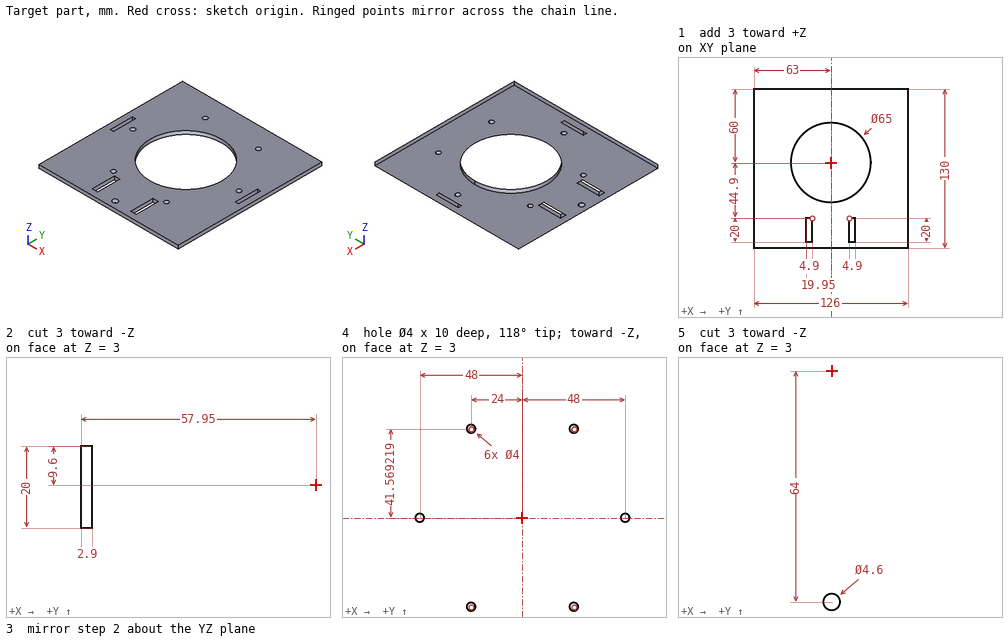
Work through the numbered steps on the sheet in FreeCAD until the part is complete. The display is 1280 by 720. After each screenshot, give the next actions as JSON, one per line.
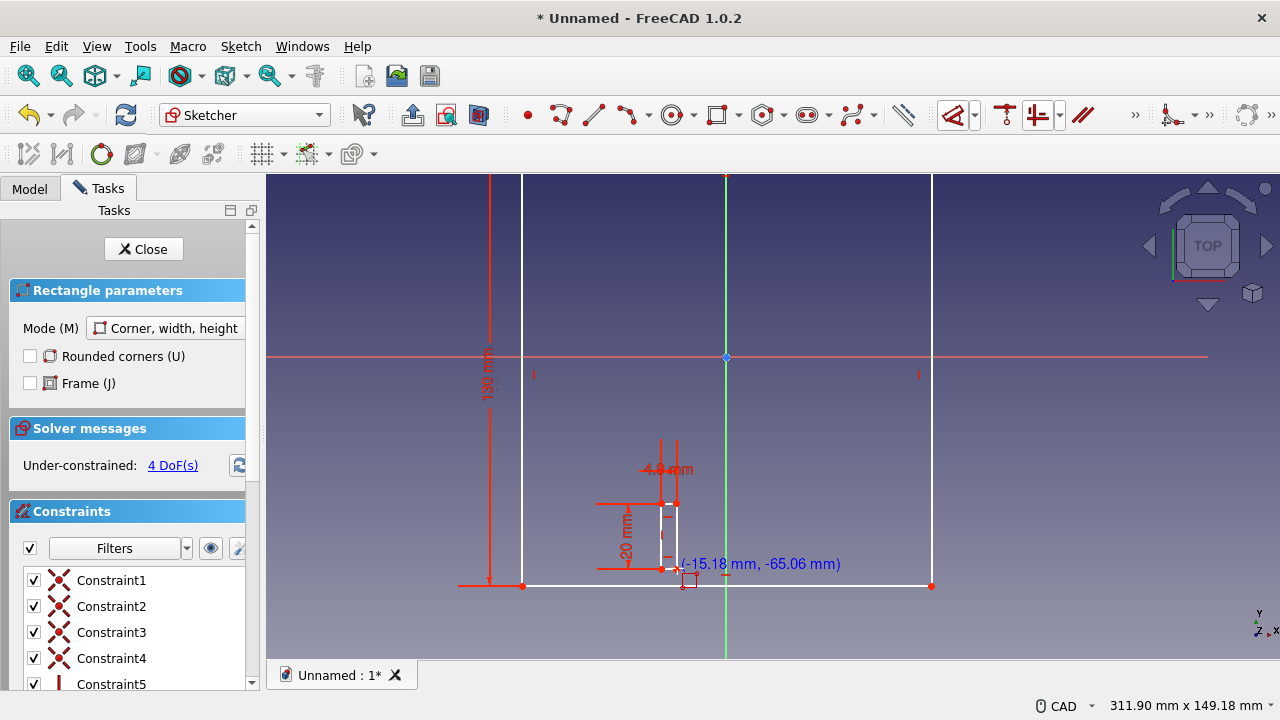
{"action": "left_click", "coordinate": [775, 503]}
{"action": "mouse_move", "coordinate": [791, 568]}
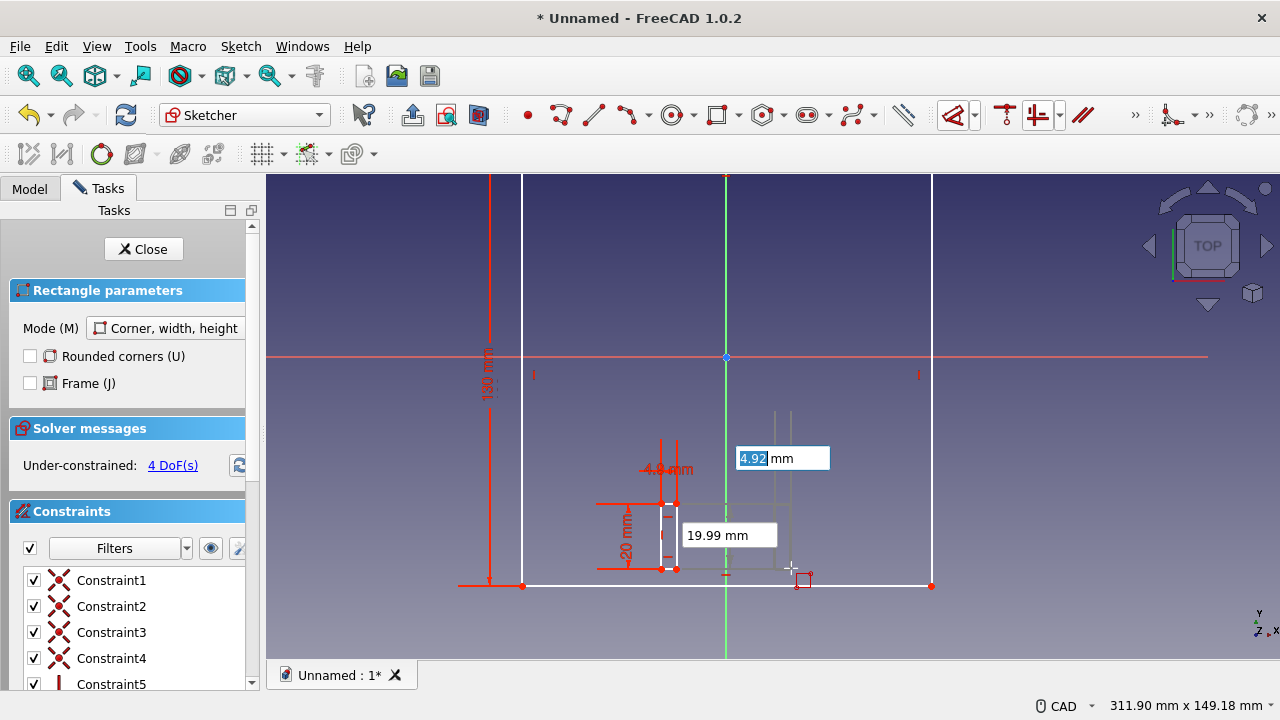
{"action": "type", "text": "4.9"}
{"action": "key", "text": "Tab"}
{"action": "type", "text": "20"}
{"action": "key", "text": "Return"}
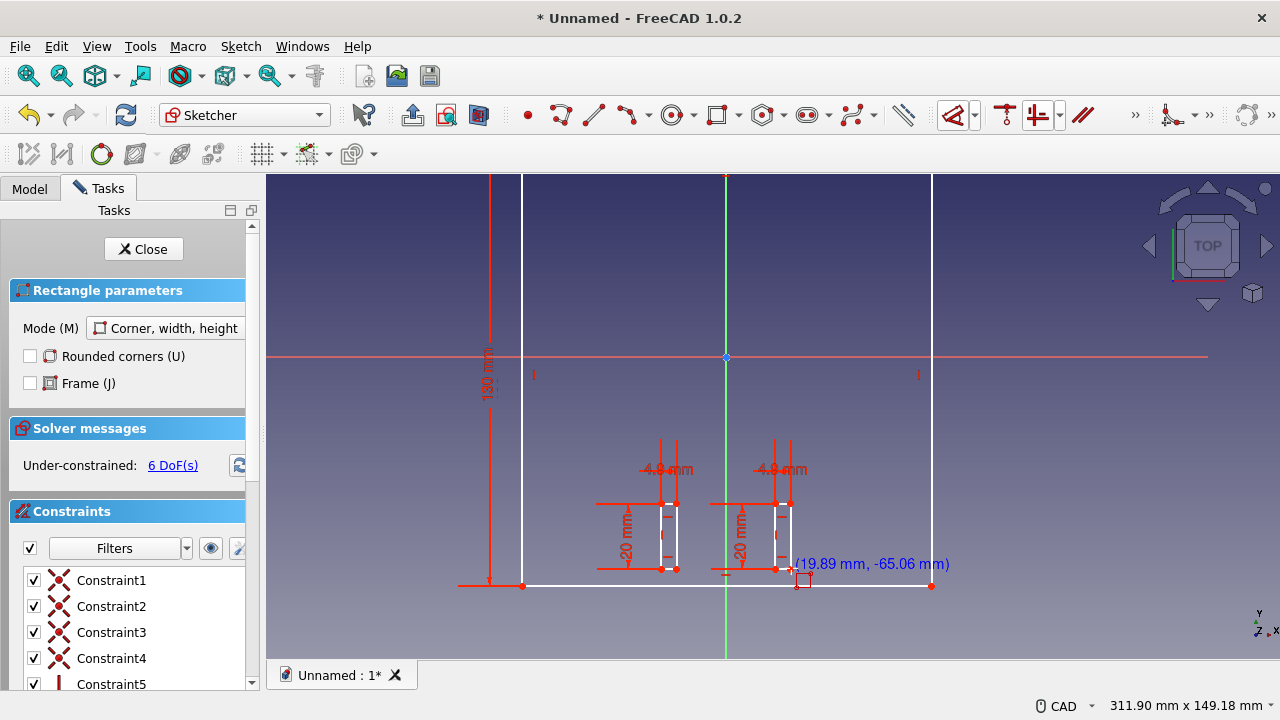
{"action": "left_click", "coordinate": [672, 116]}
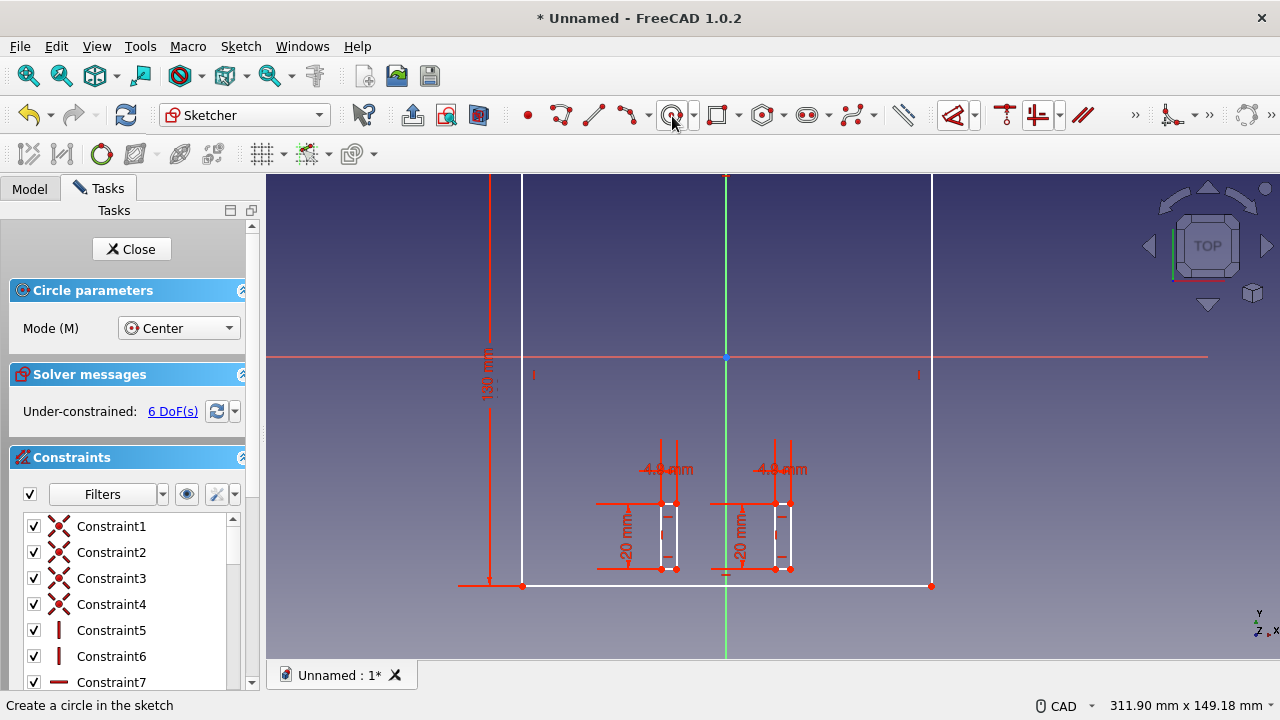
{"action": "left_click", "coordinate": [726, 357]}
{"action": "mouse_move", "coordinate": [801, 283]}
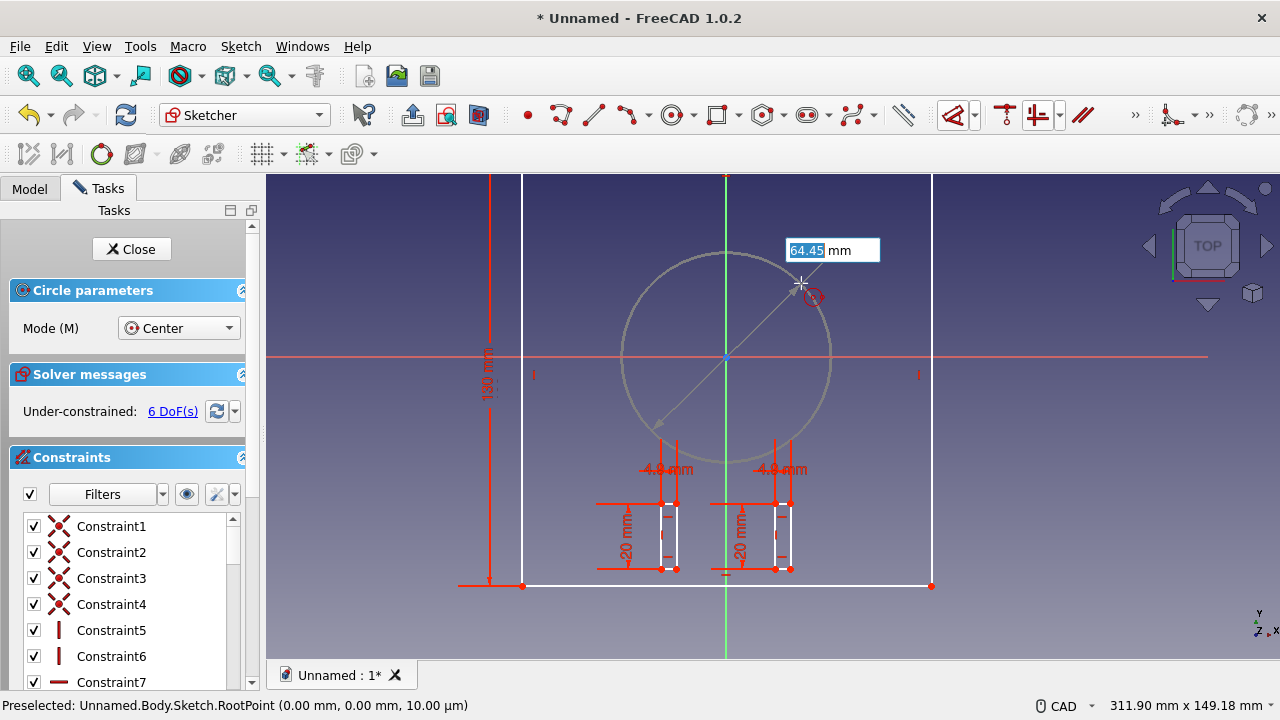
{"action": "type", "text": "65"}
{"action": "key", "text": "Return"}
{"action": "key", "text": "Escape"}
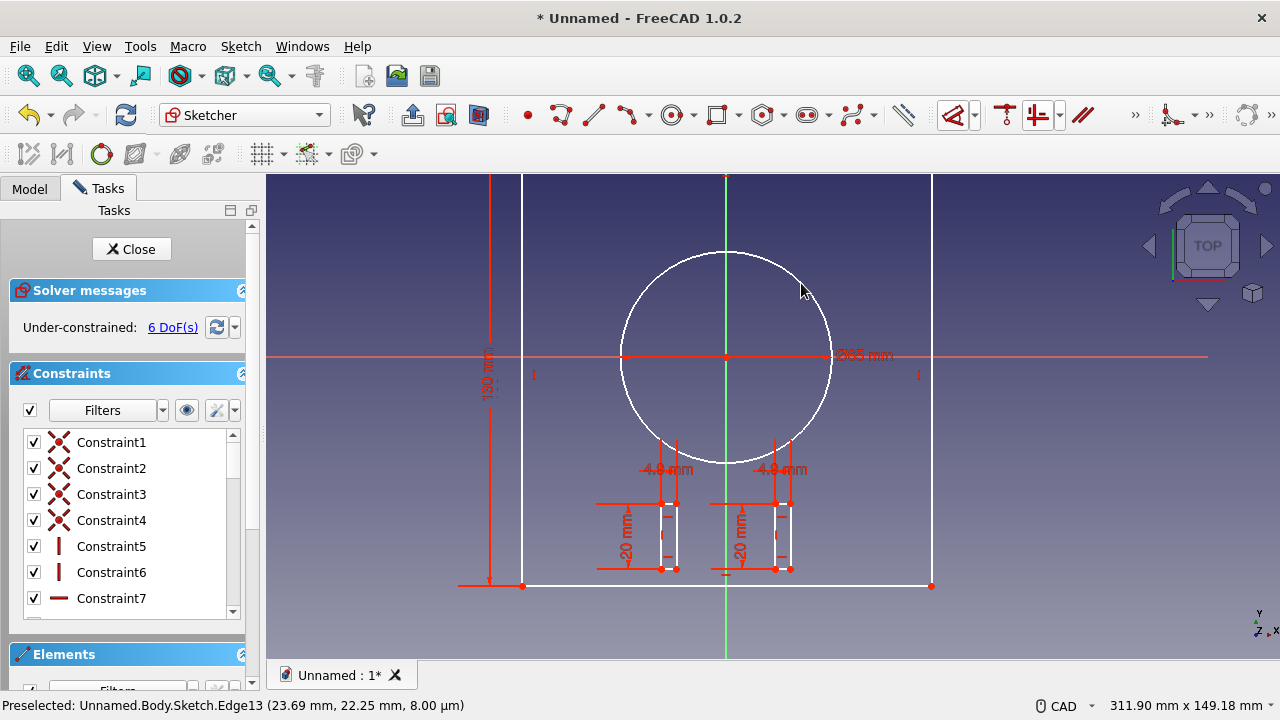
{"action": "left_click", "coordinate": [677, 504]}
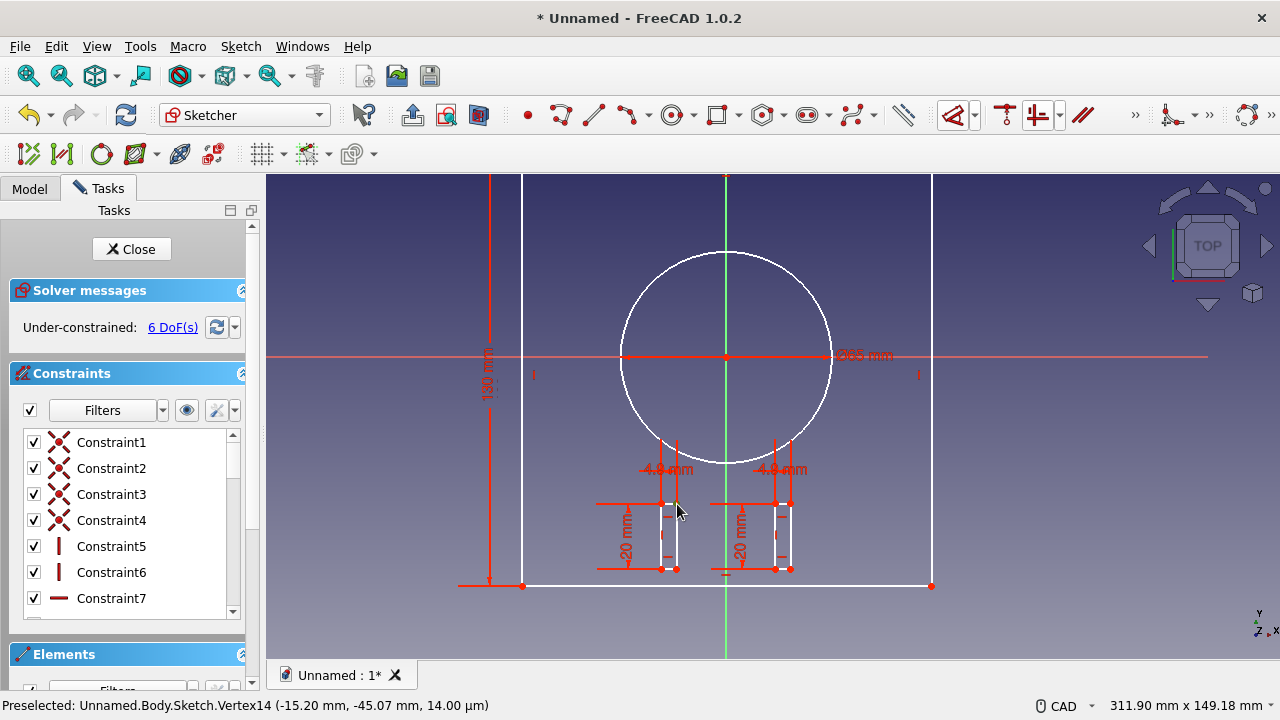
{"action": "left_click", "coordinate": [775, 504]}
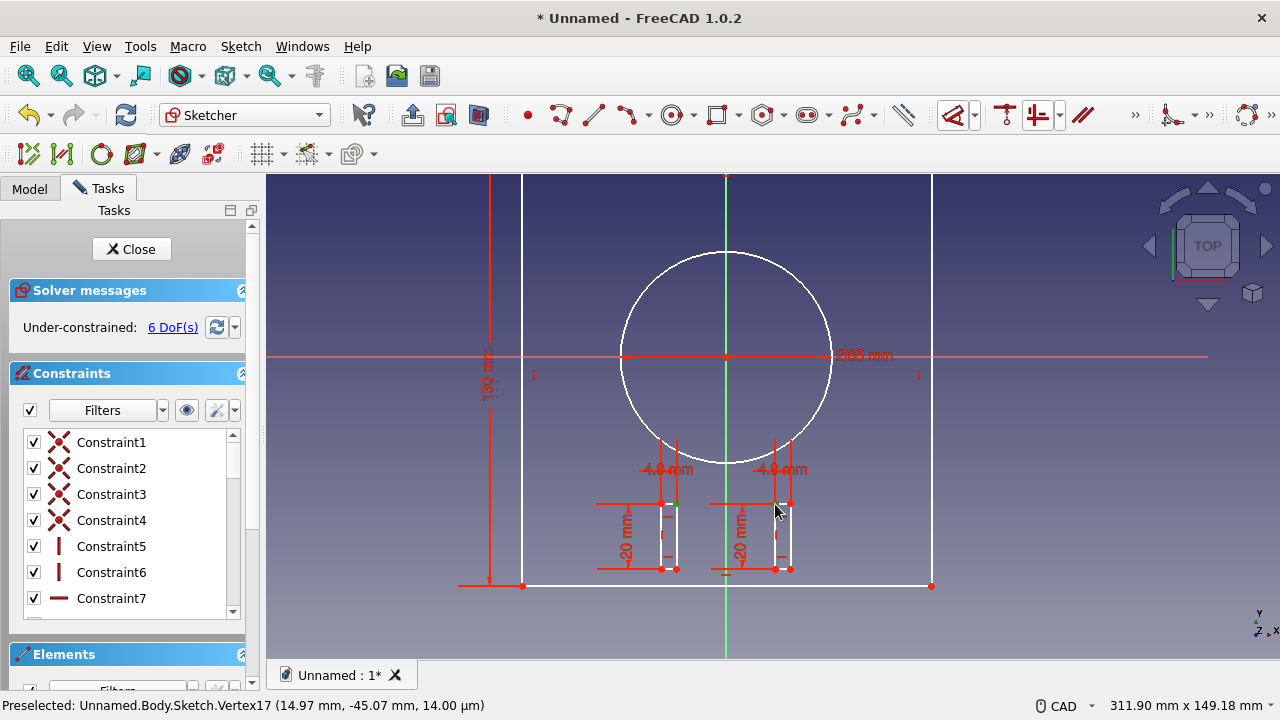
{"action": "left_click", "coordinate": [726, 539]}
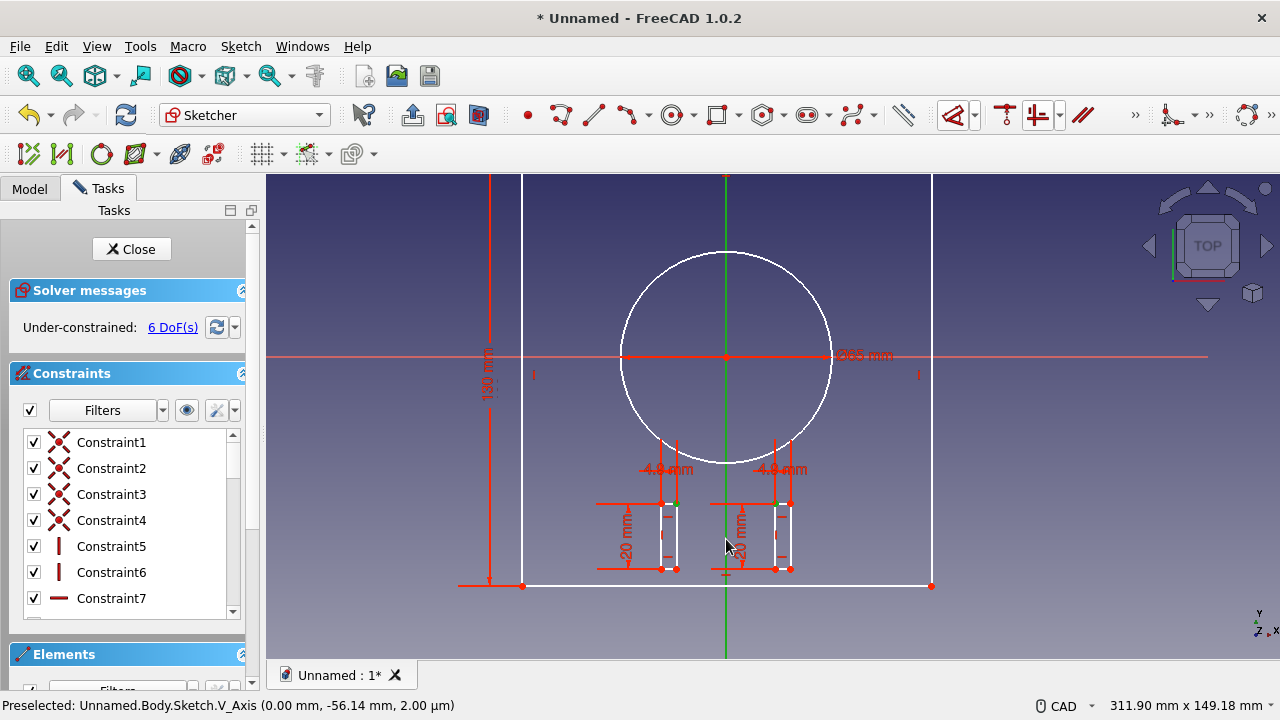
{"action": "key", "text": "s"}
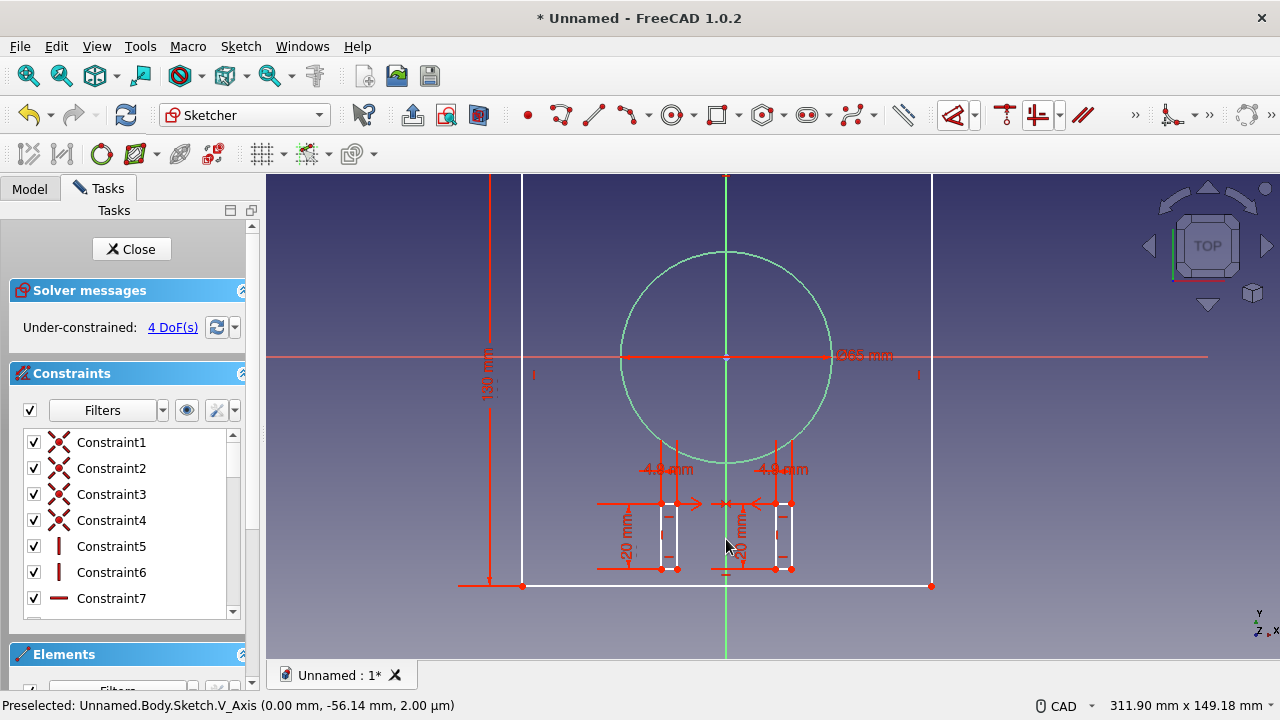
{"action": "left_click", "coordinate": [952, 116]}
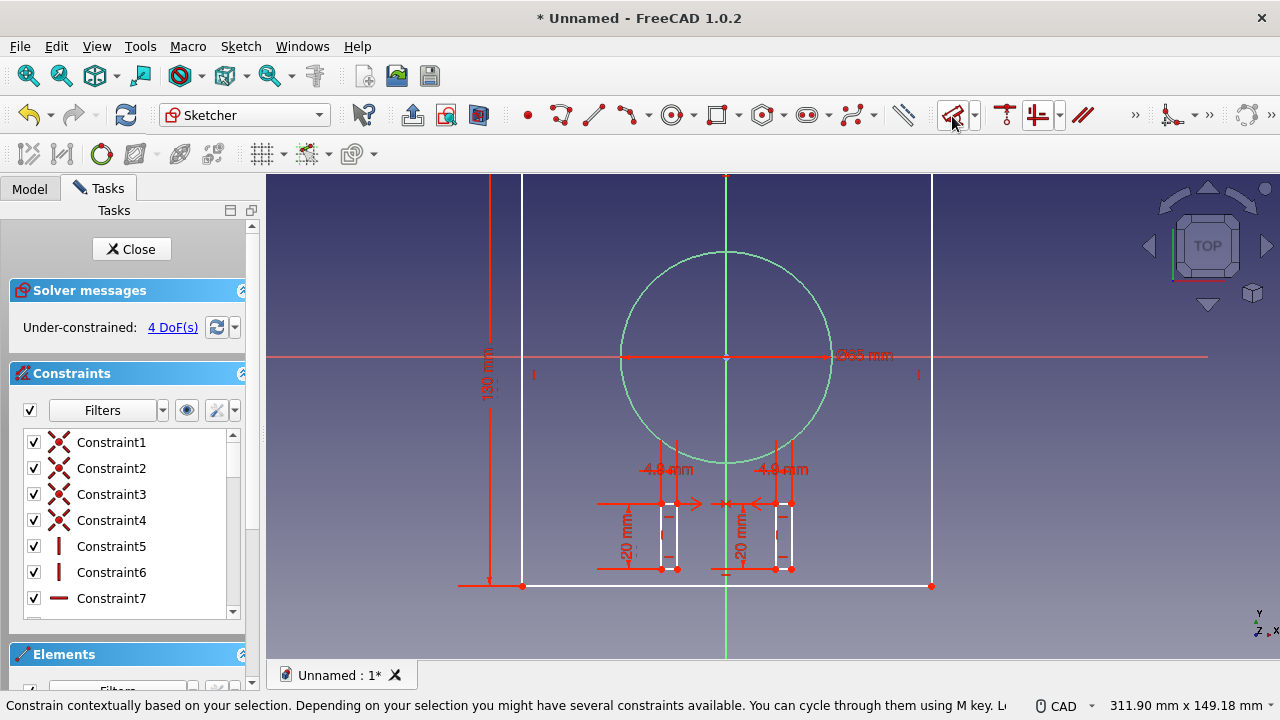
{"action": "scroll", "coordinate": [660, 503], "scroll_direction": "down", "scroll_amount": 2}